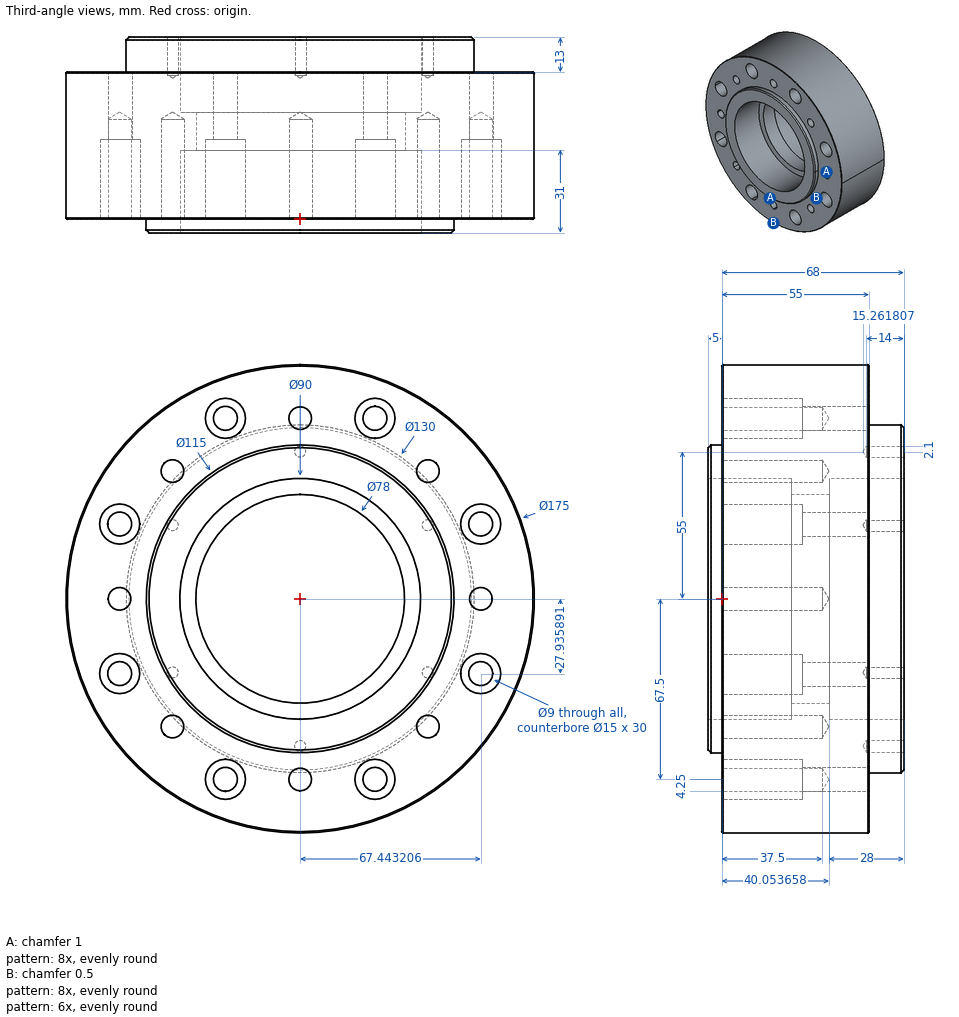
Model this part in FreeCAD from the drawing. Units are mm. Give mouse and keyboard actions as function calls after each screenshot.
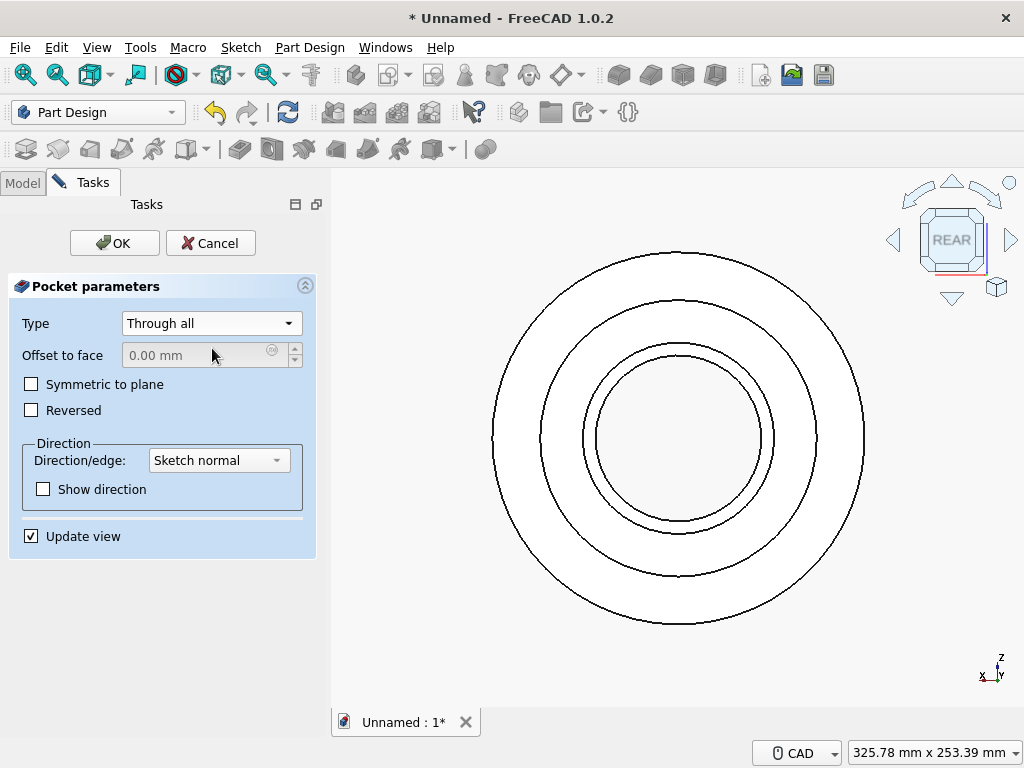
click(115, 243)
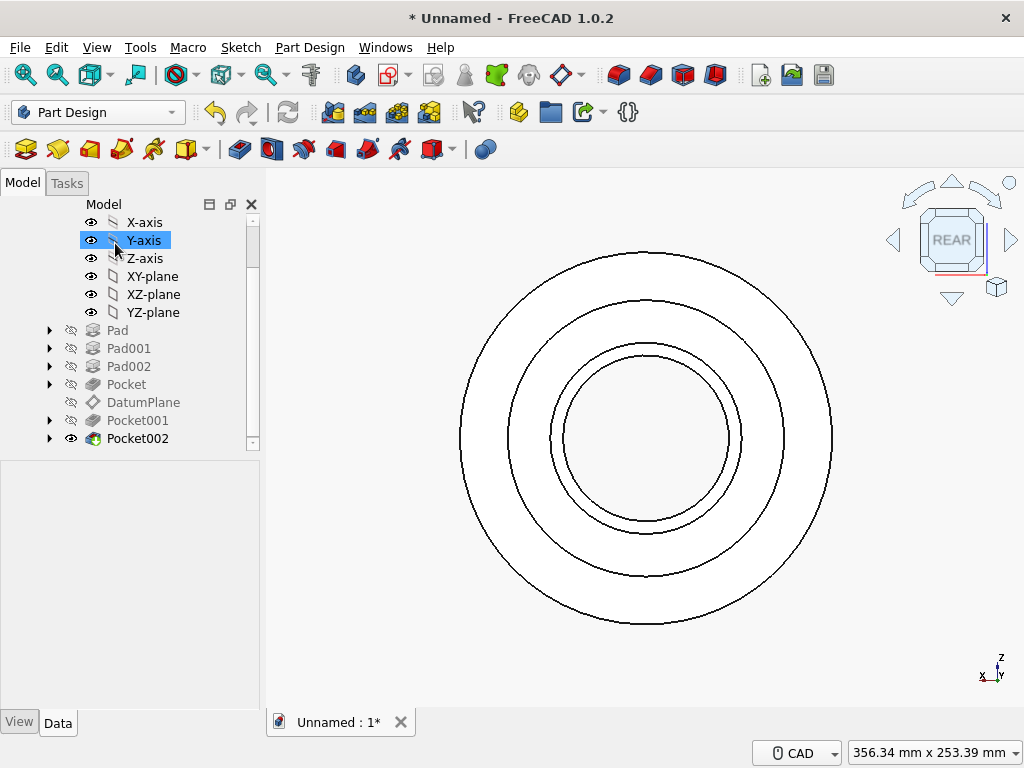
click(784, 437)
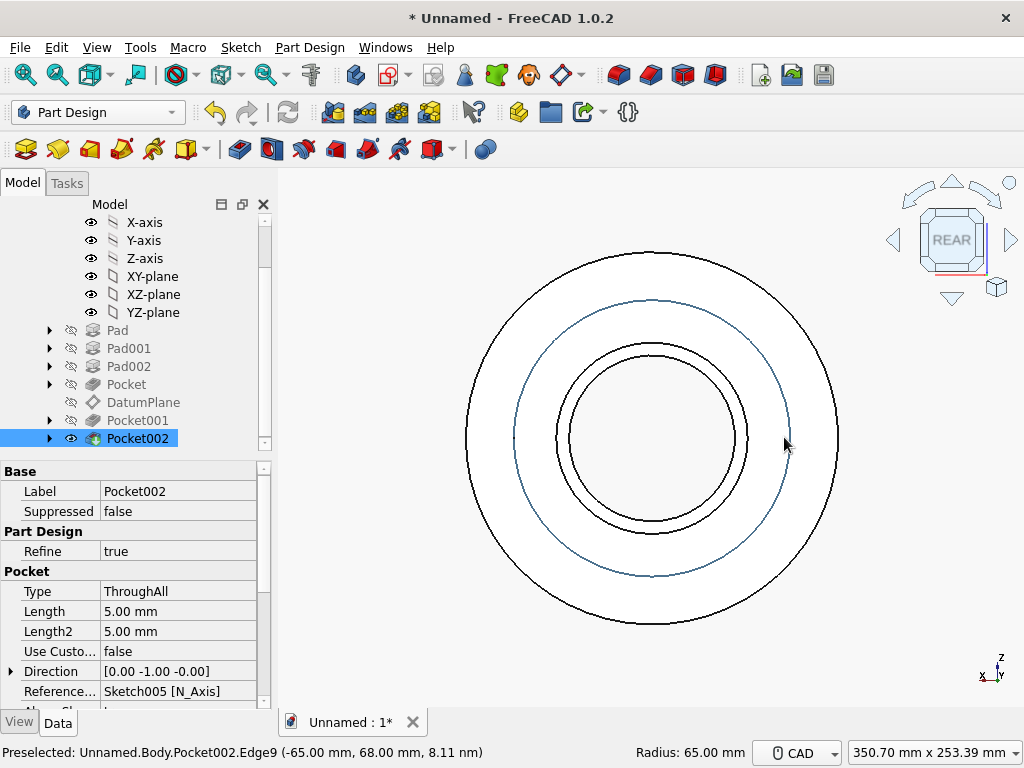
key(0)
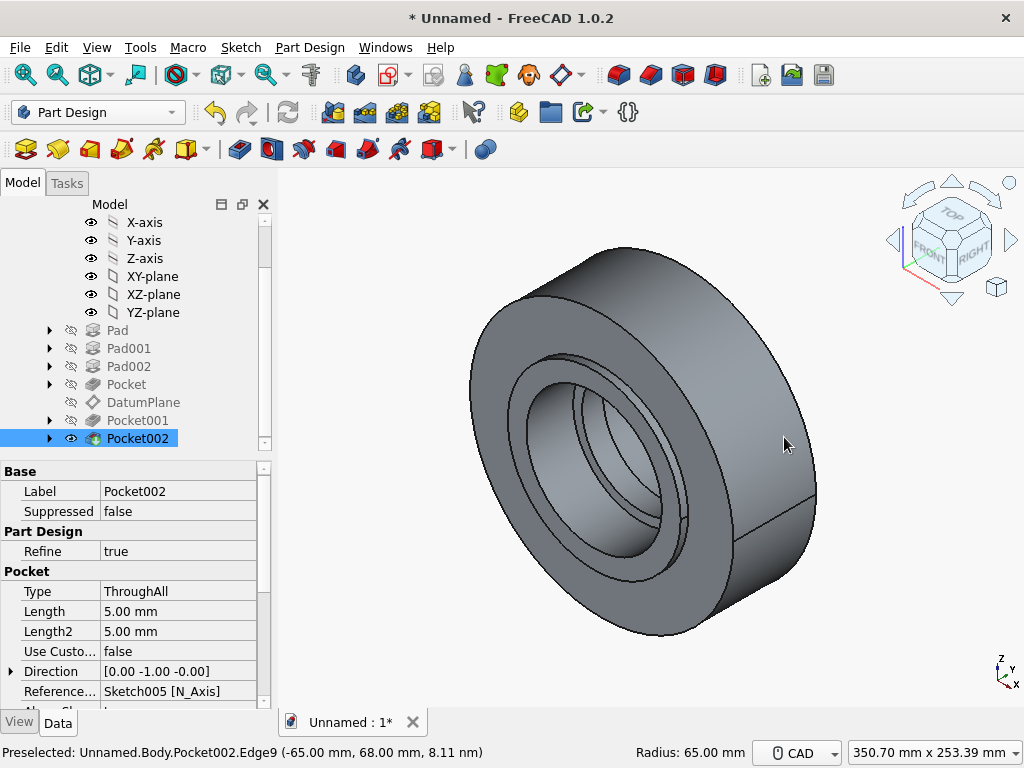
click(567, 359, ctrl)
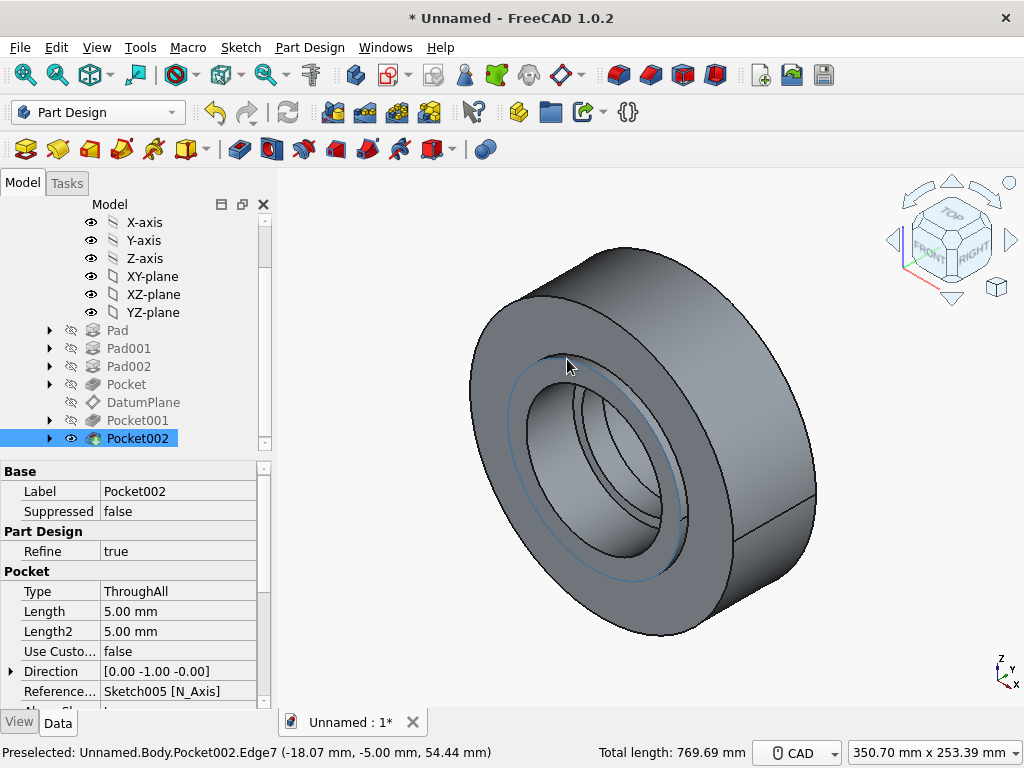
click(652, 76)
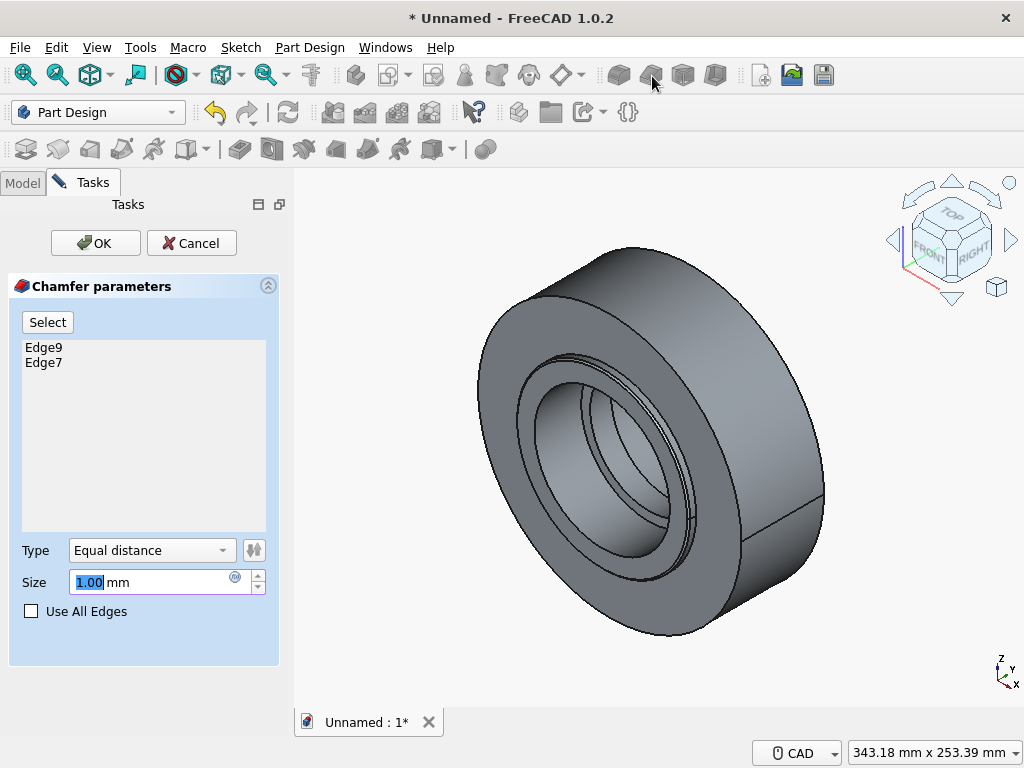
text(1)
key(Tab)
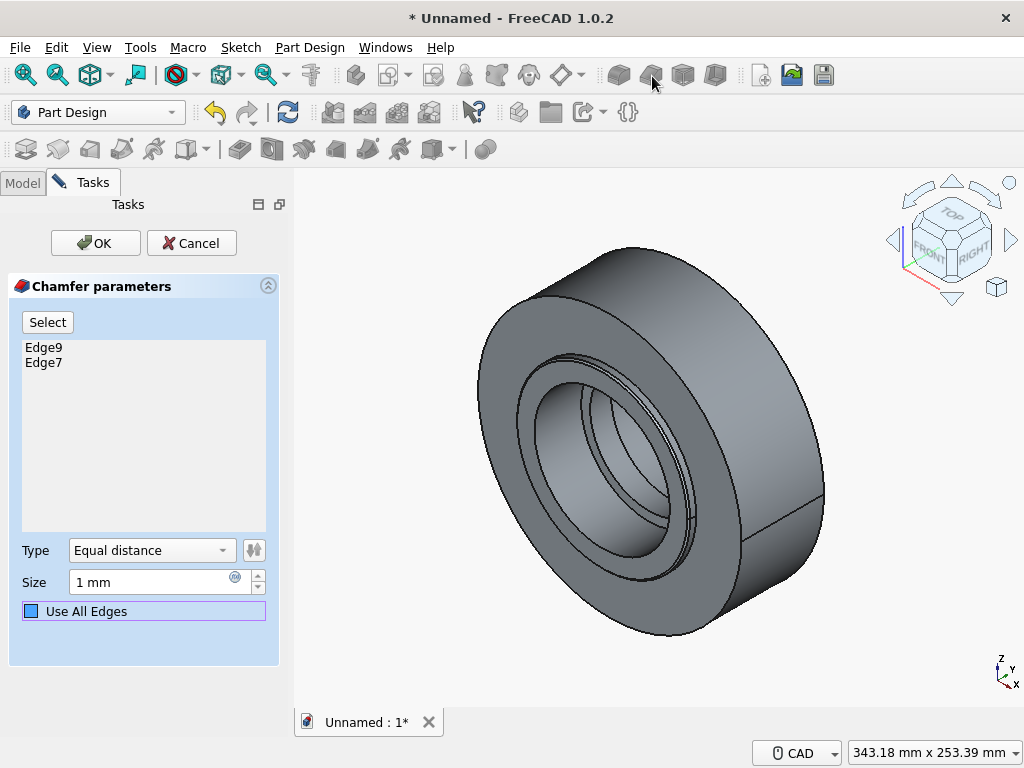
click(96, 243)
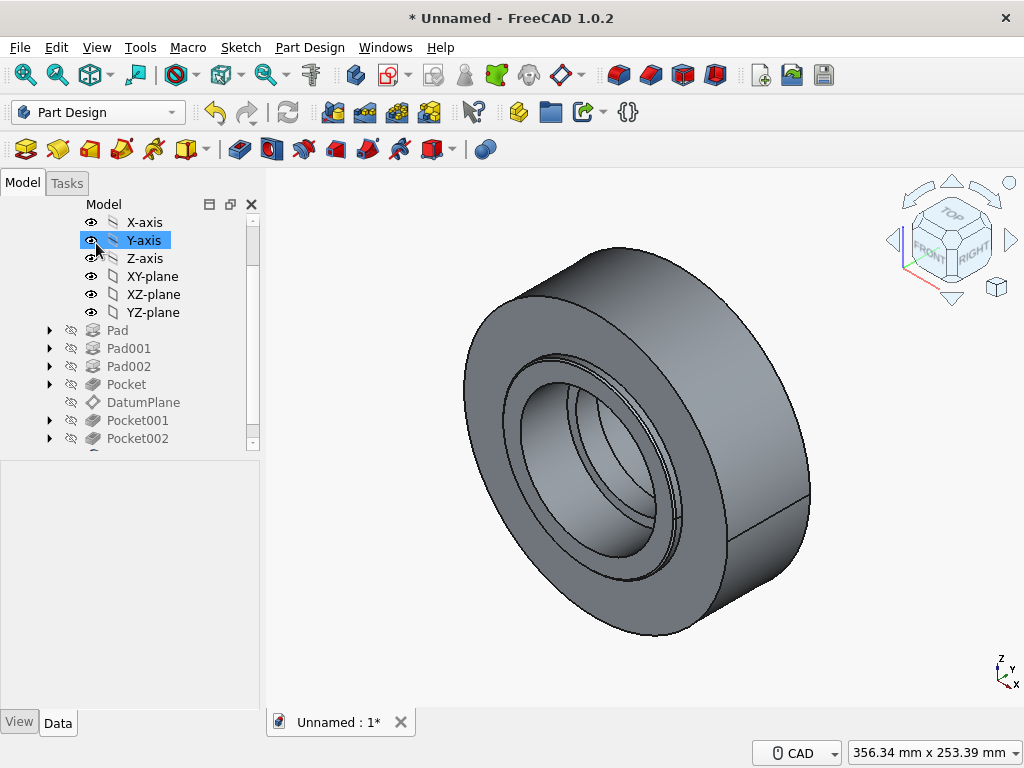
click(388, 76)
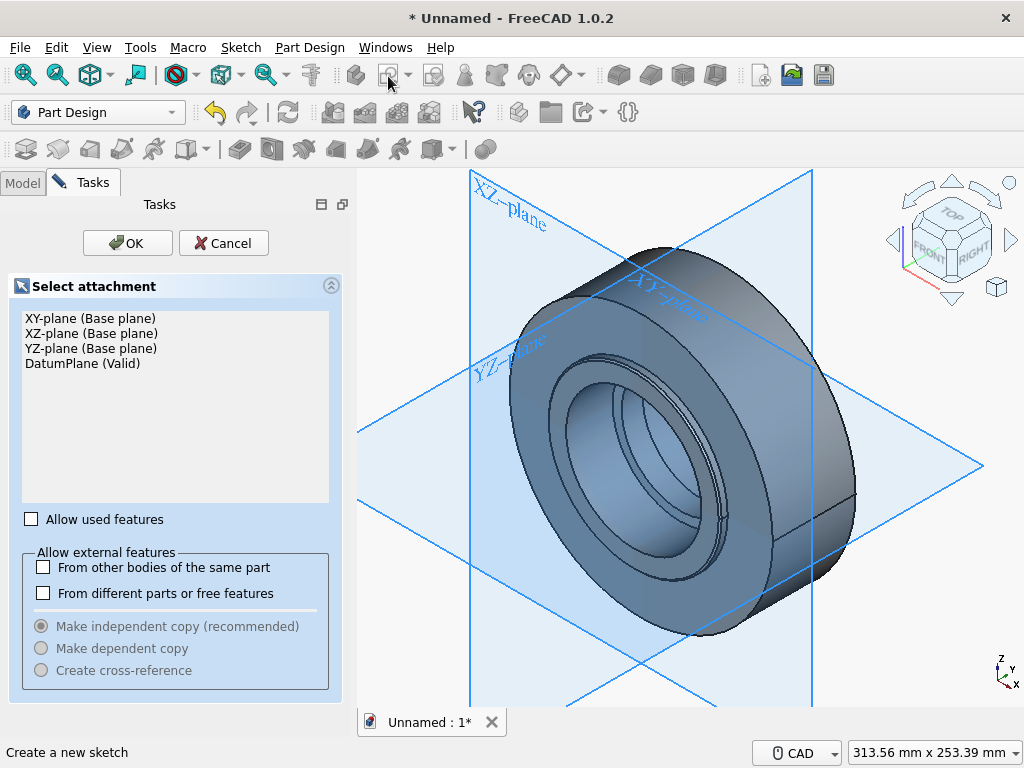
click(82, 334)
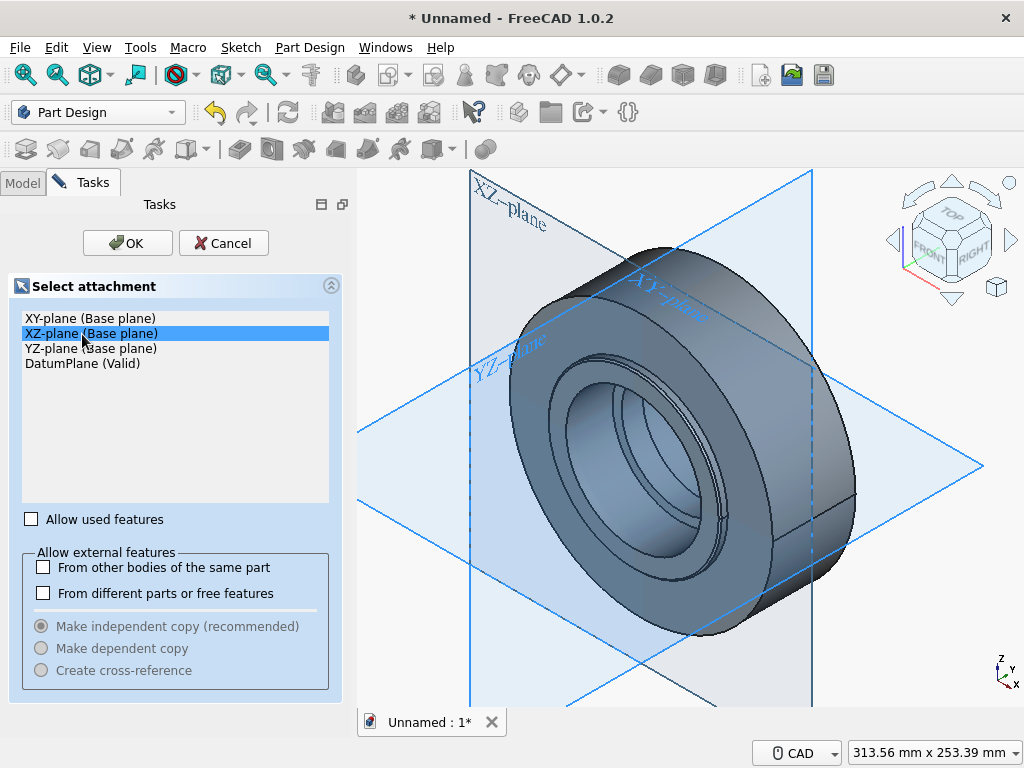
click(128, 243)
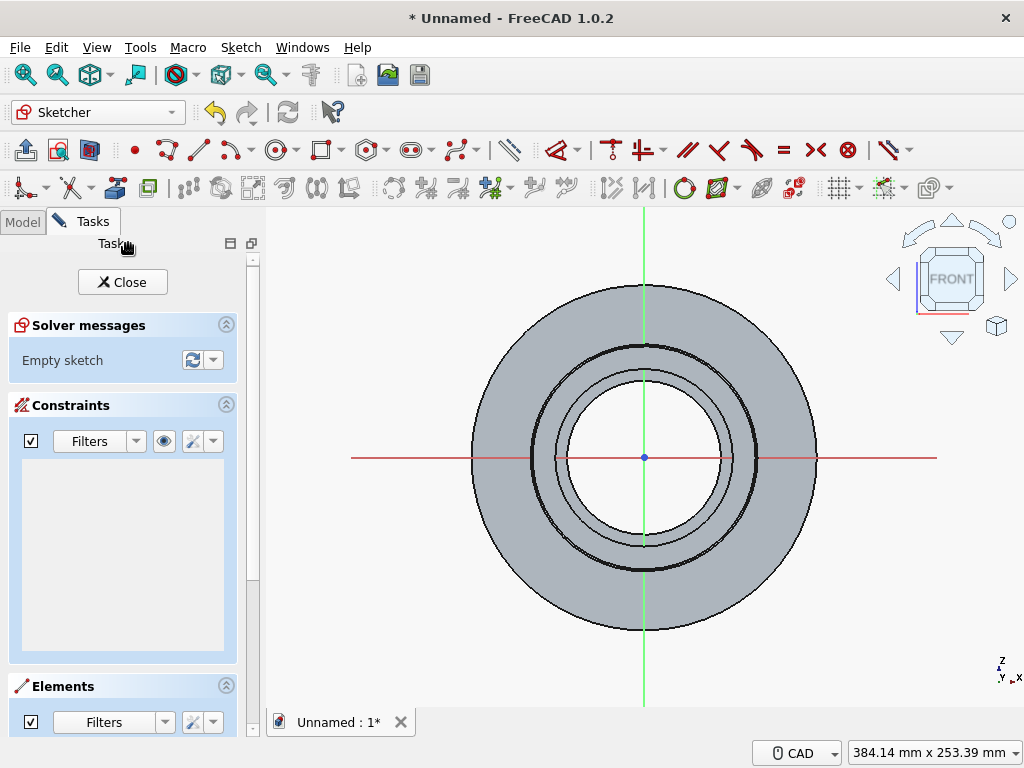
click(90, 150)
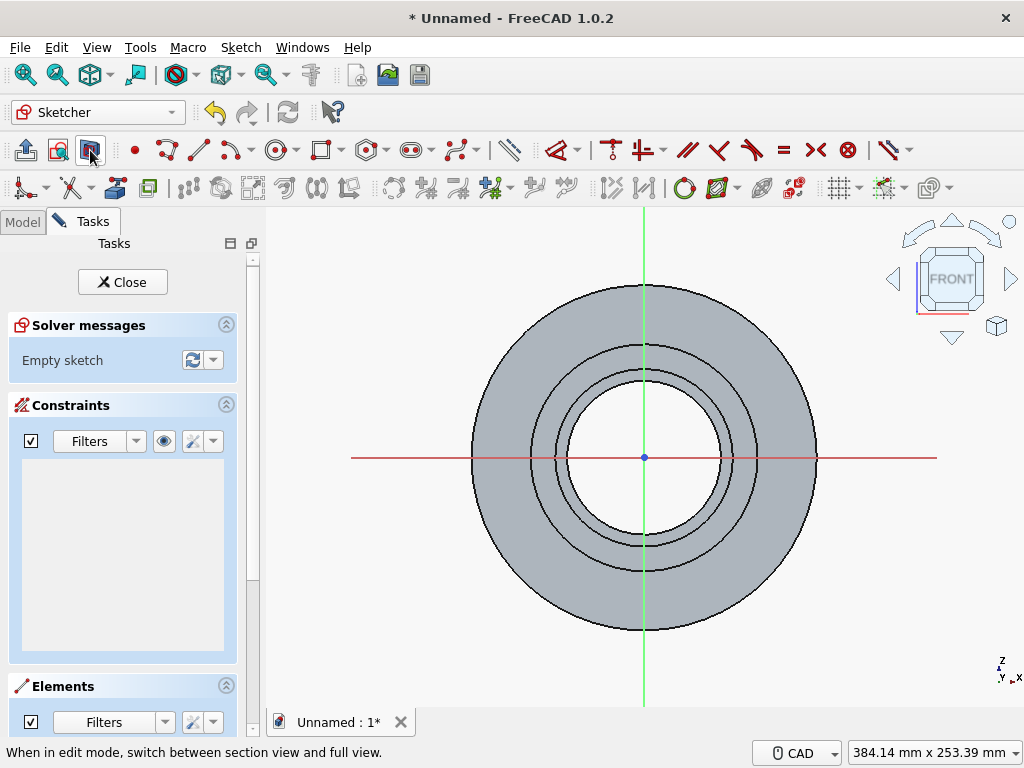
scroll(790, 517, up, 14)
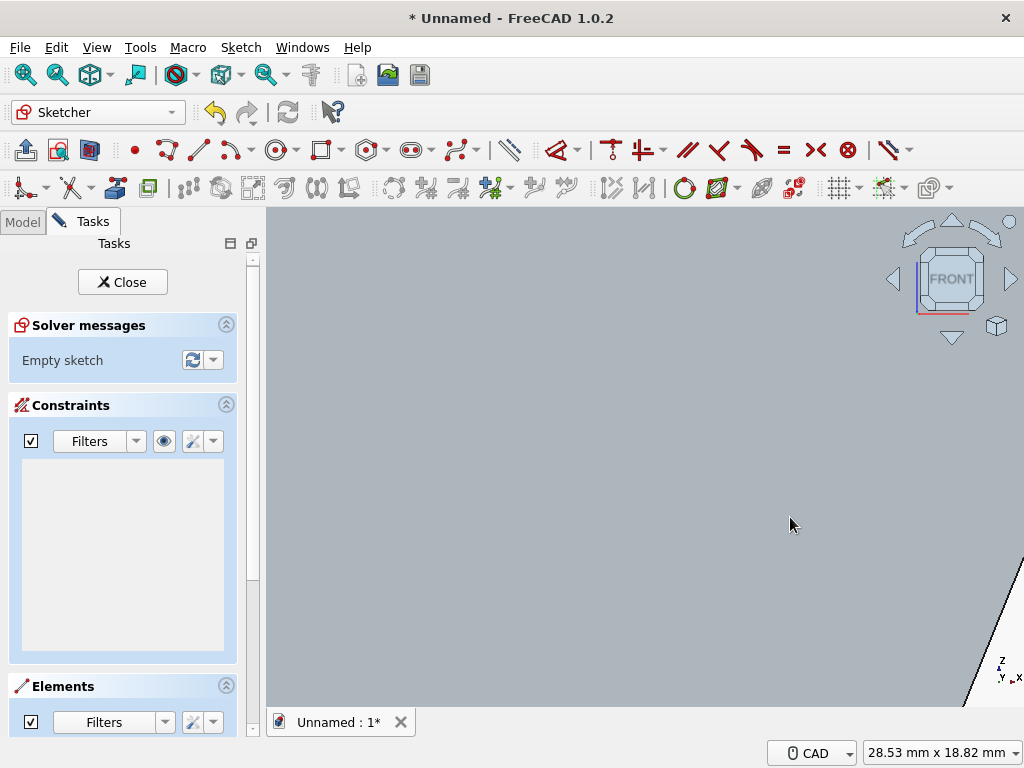
click(276, 150)